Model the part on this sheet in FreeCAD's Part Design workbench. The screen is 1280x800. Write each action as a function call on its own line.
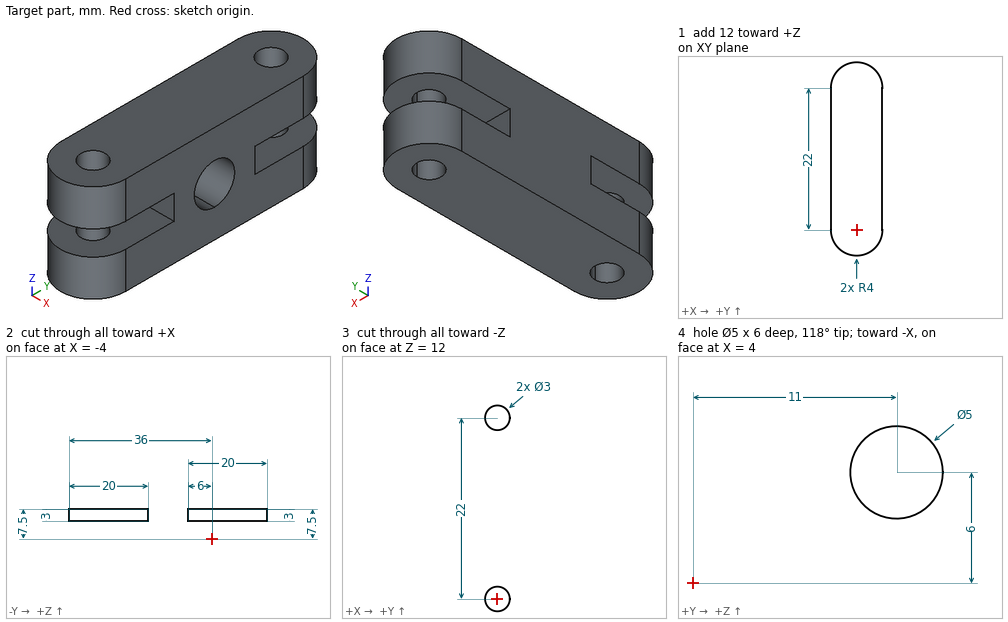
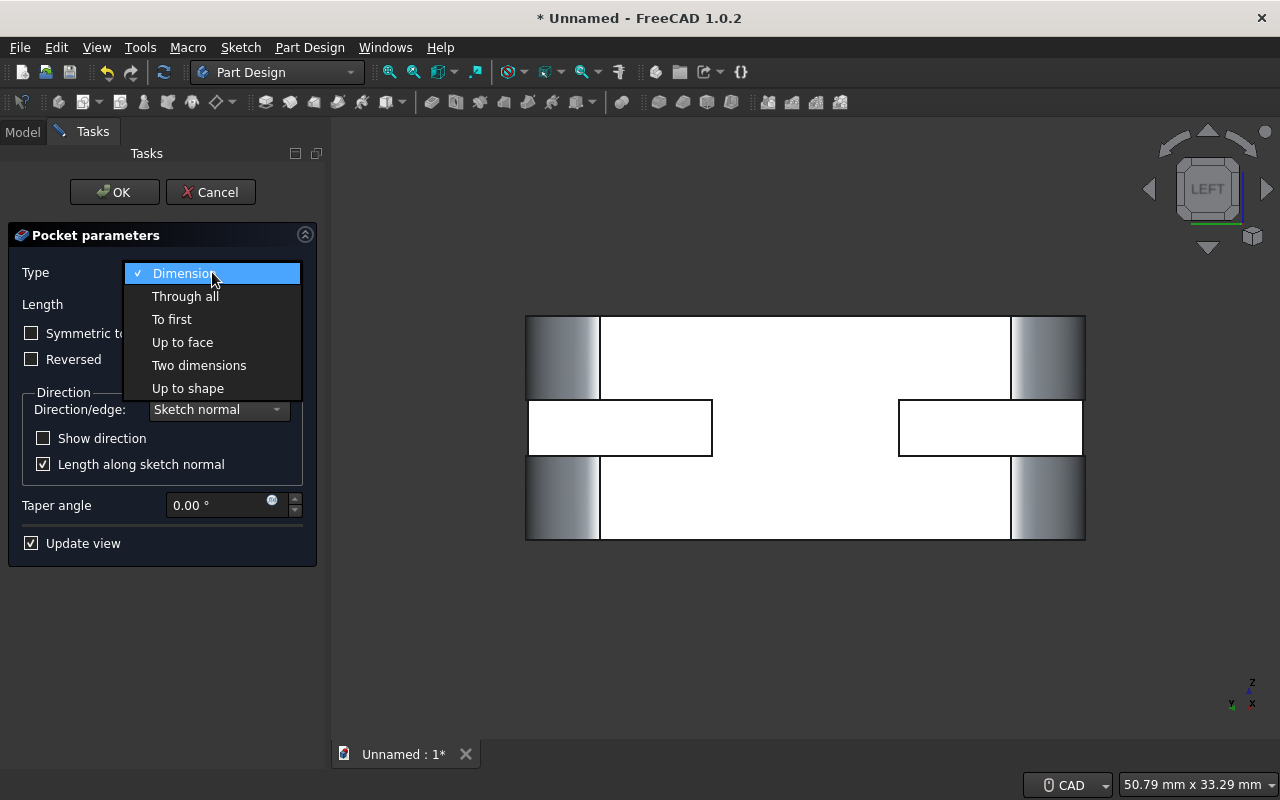
click(212, 296)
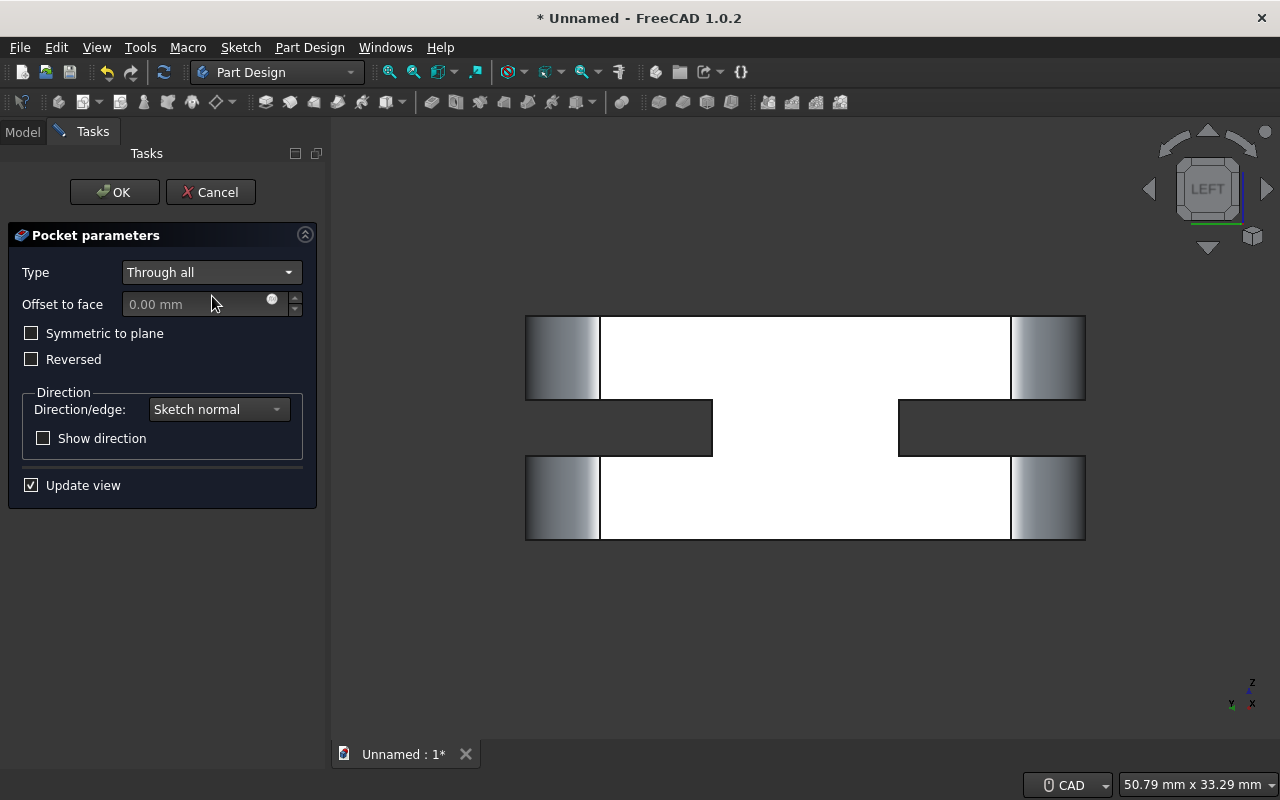
click(115, 192)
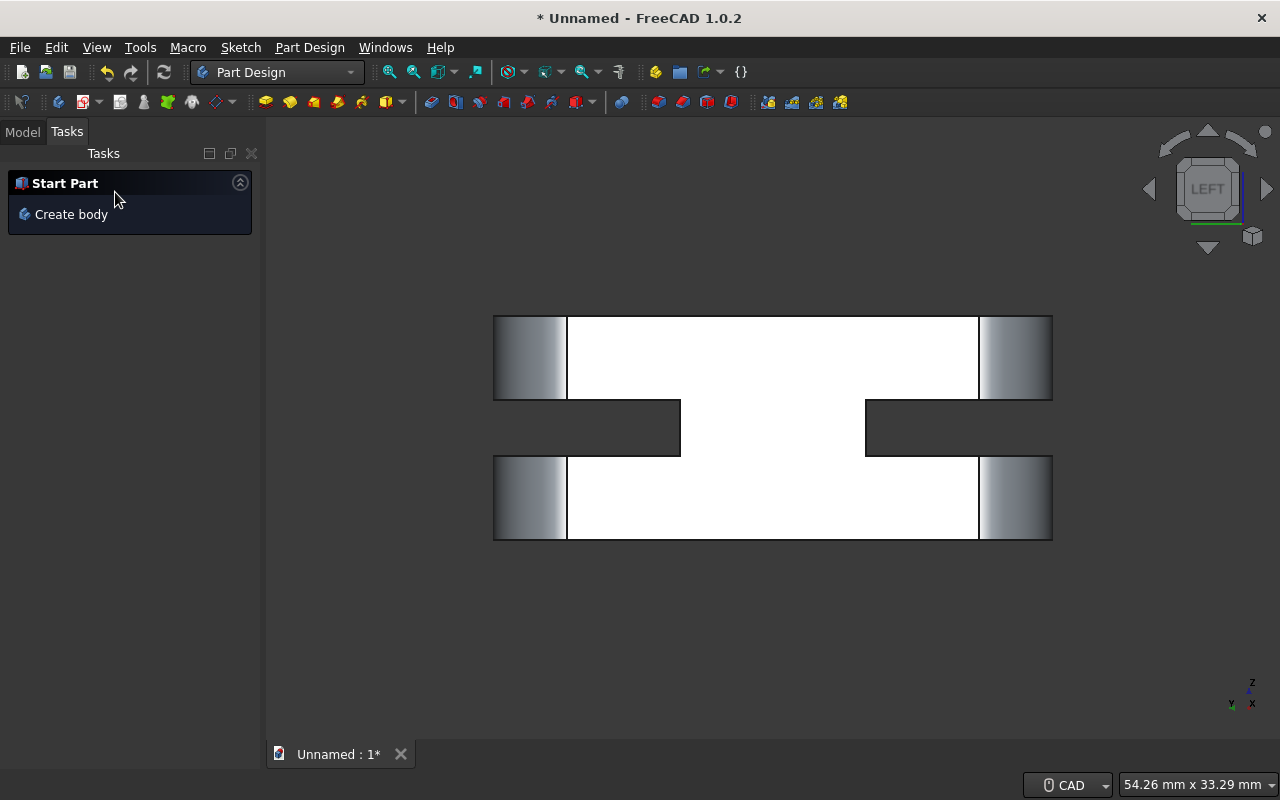
key(0)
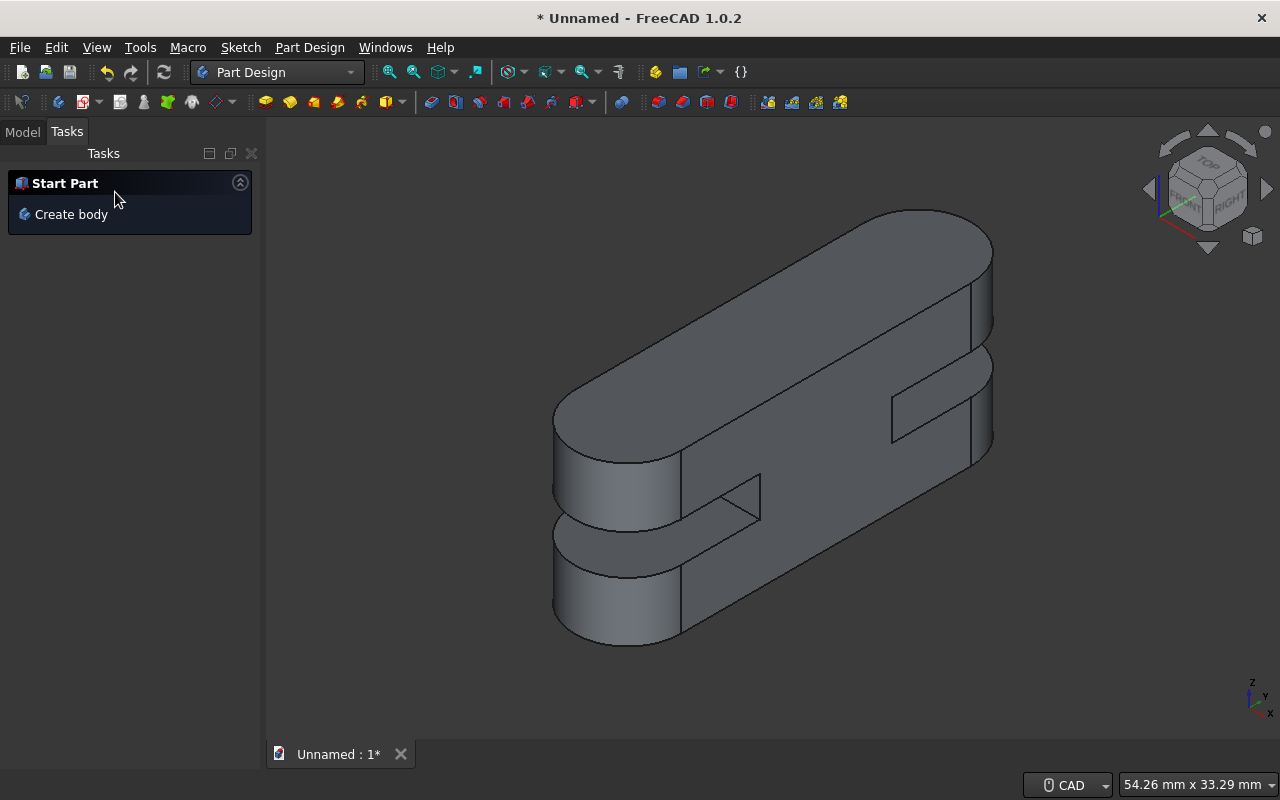
click(886, 270)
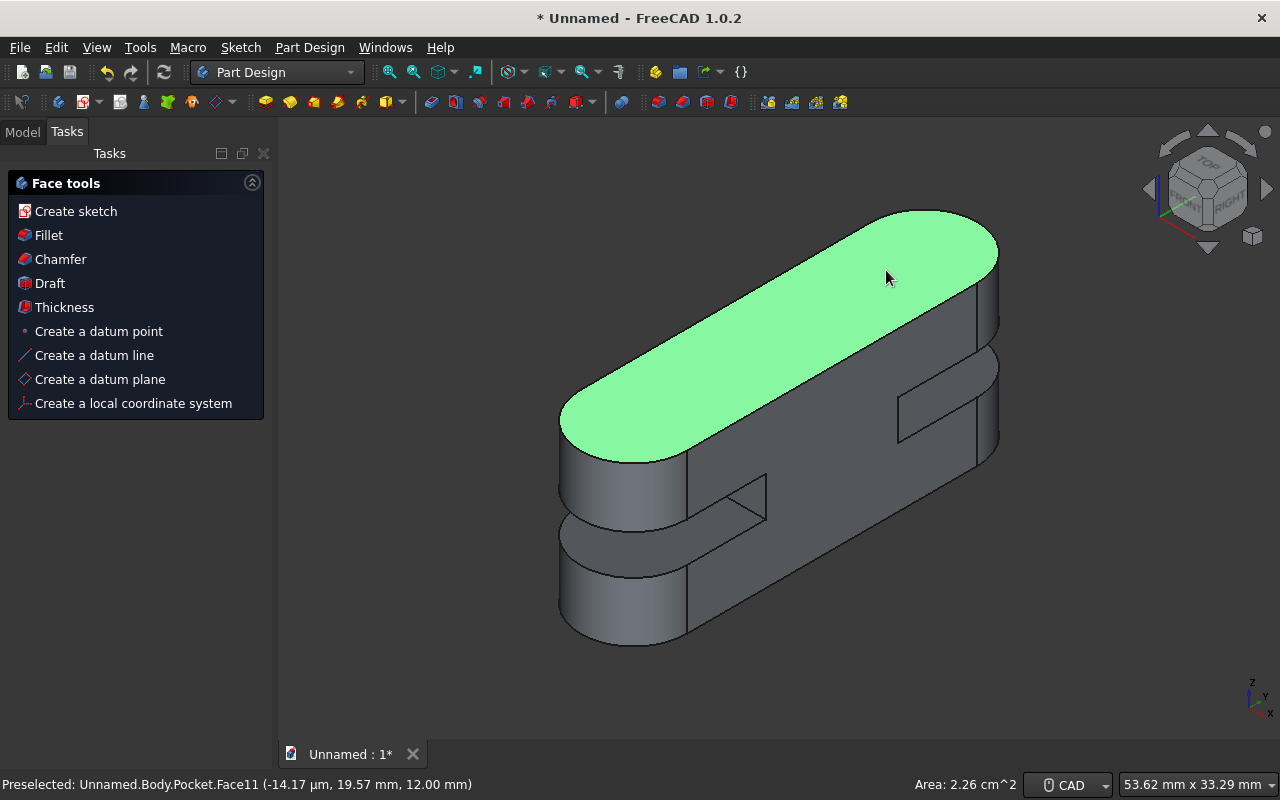
click(84, 102)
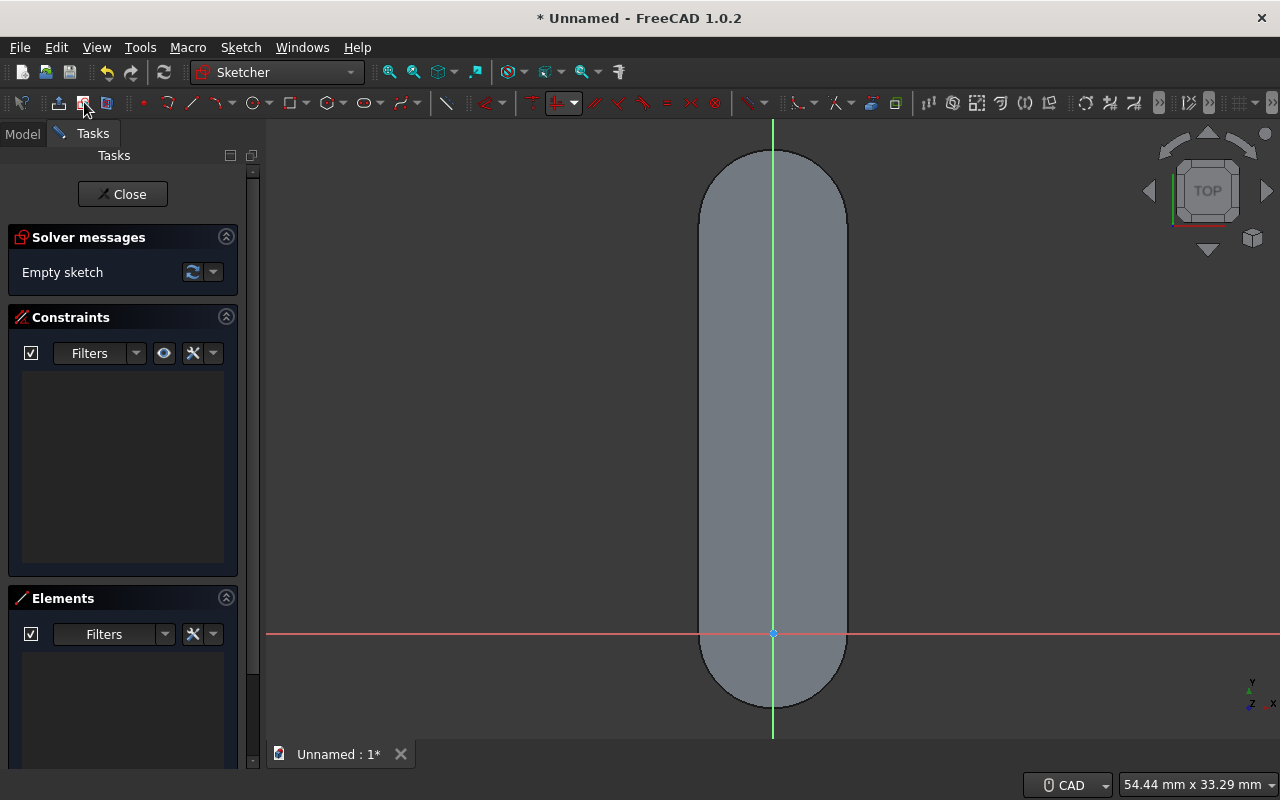
click(254, 104)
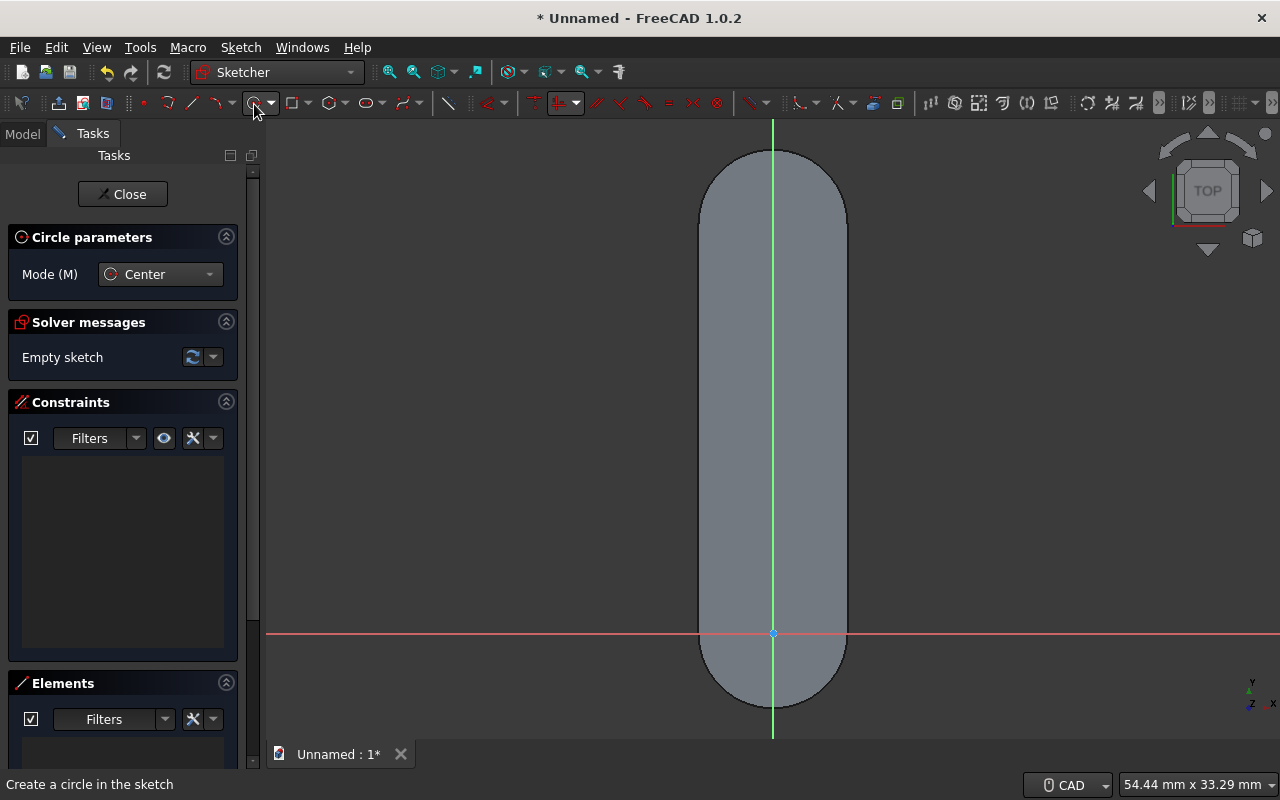
click(773, 224)
move(793, 204)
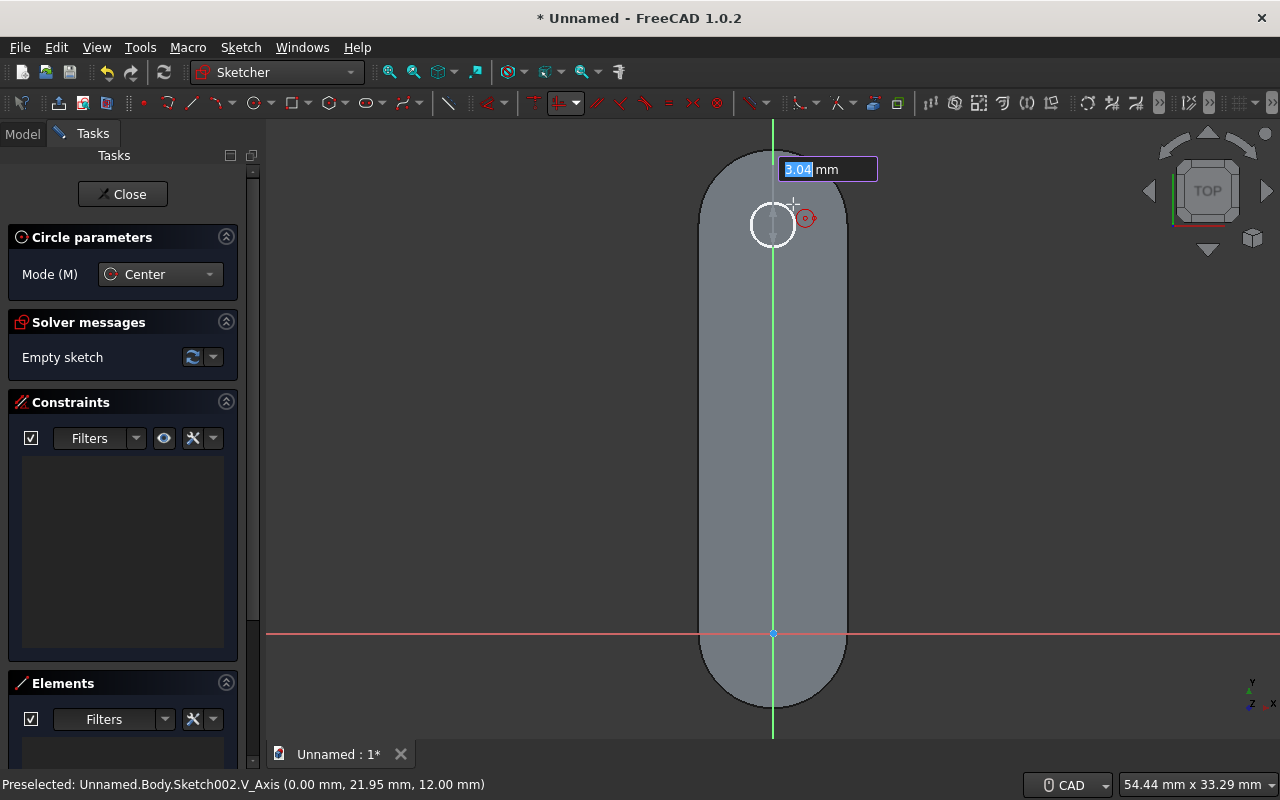
text(3)
key(Return)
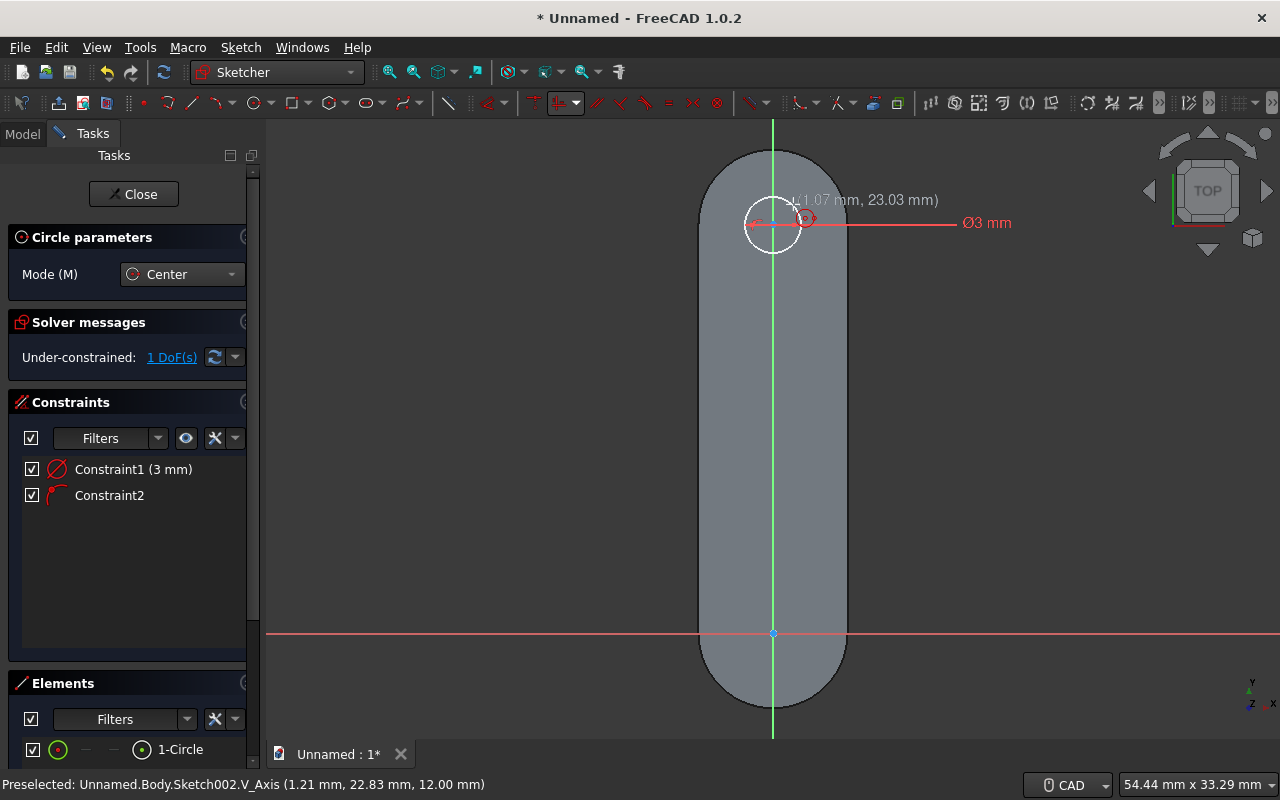
click(773, 634)
move(793, 614)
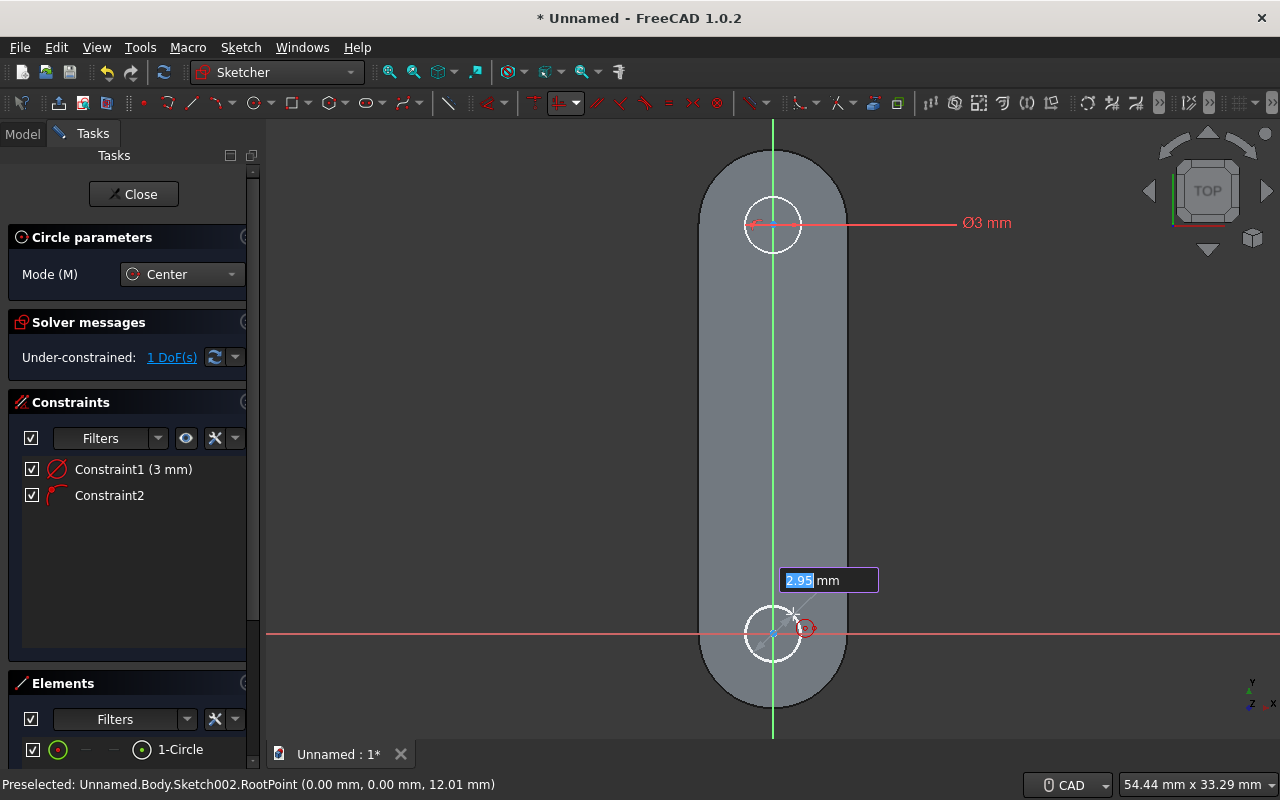
text(3)
key(Return)
key(Escape)